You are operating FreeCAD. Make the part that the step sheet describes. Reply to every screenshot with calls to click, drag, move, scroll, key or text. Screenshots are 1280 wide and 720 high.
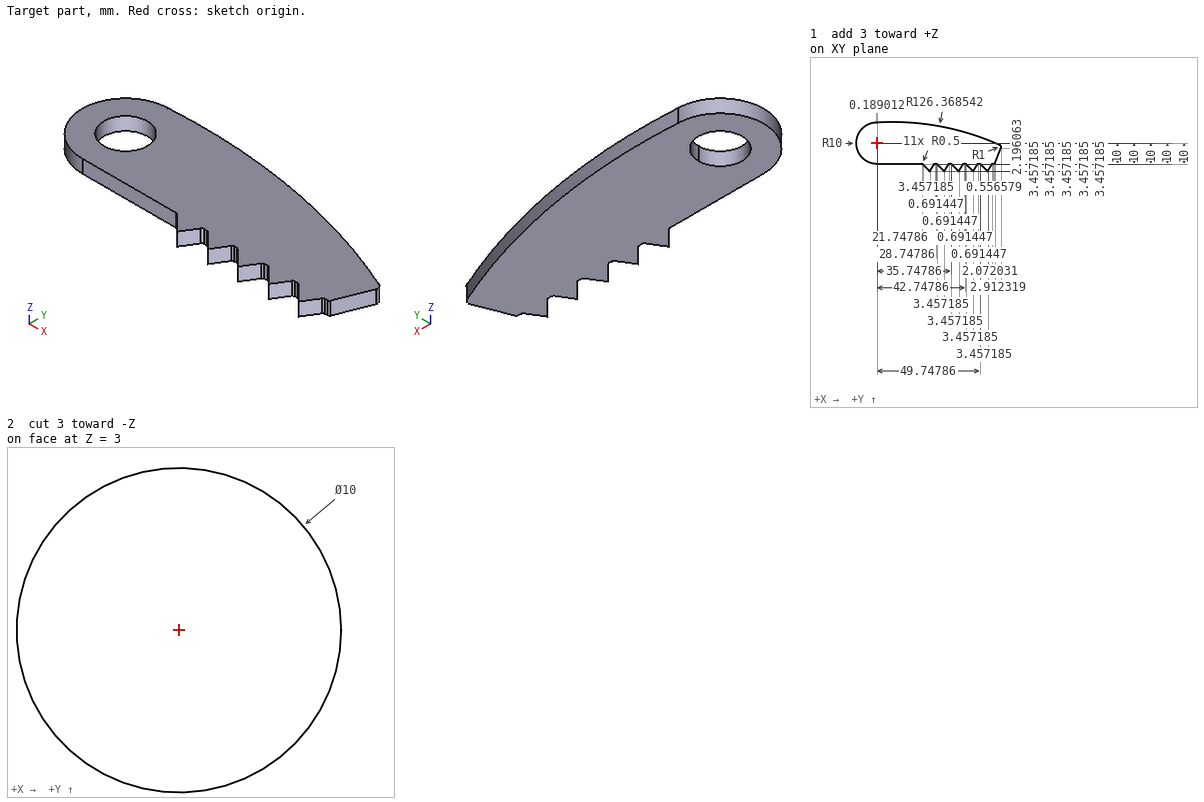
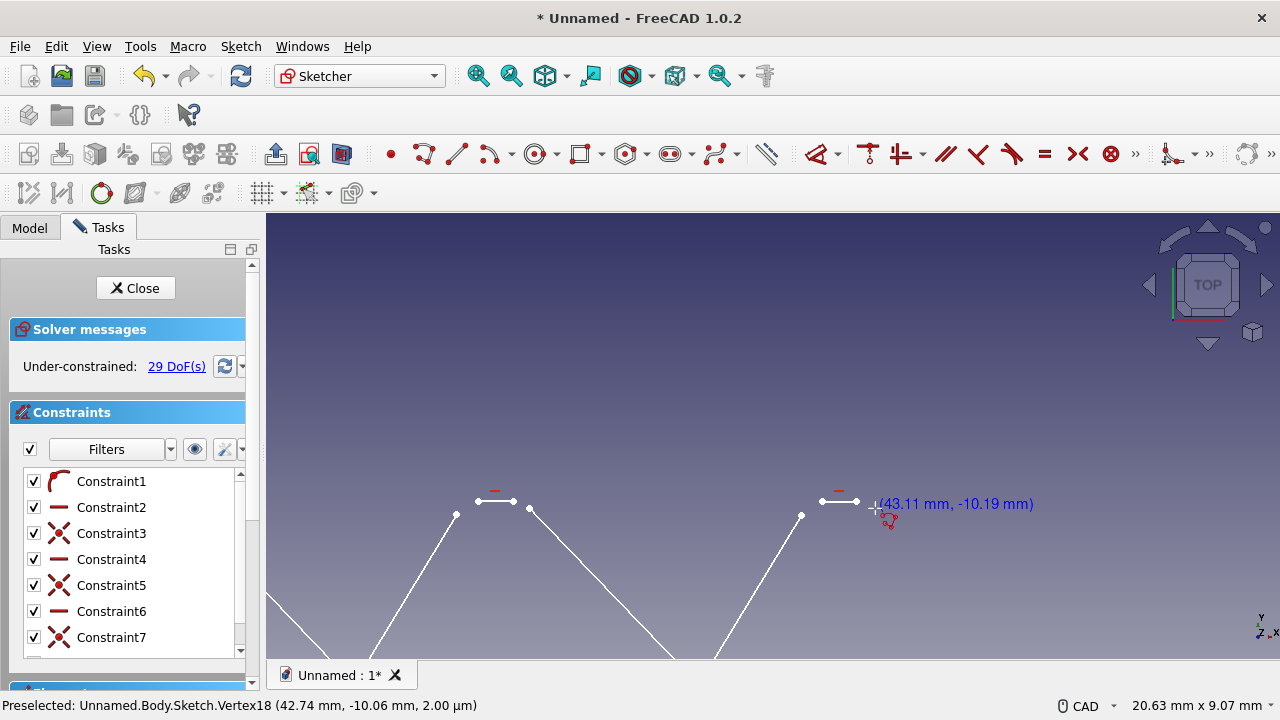
click(874, 507)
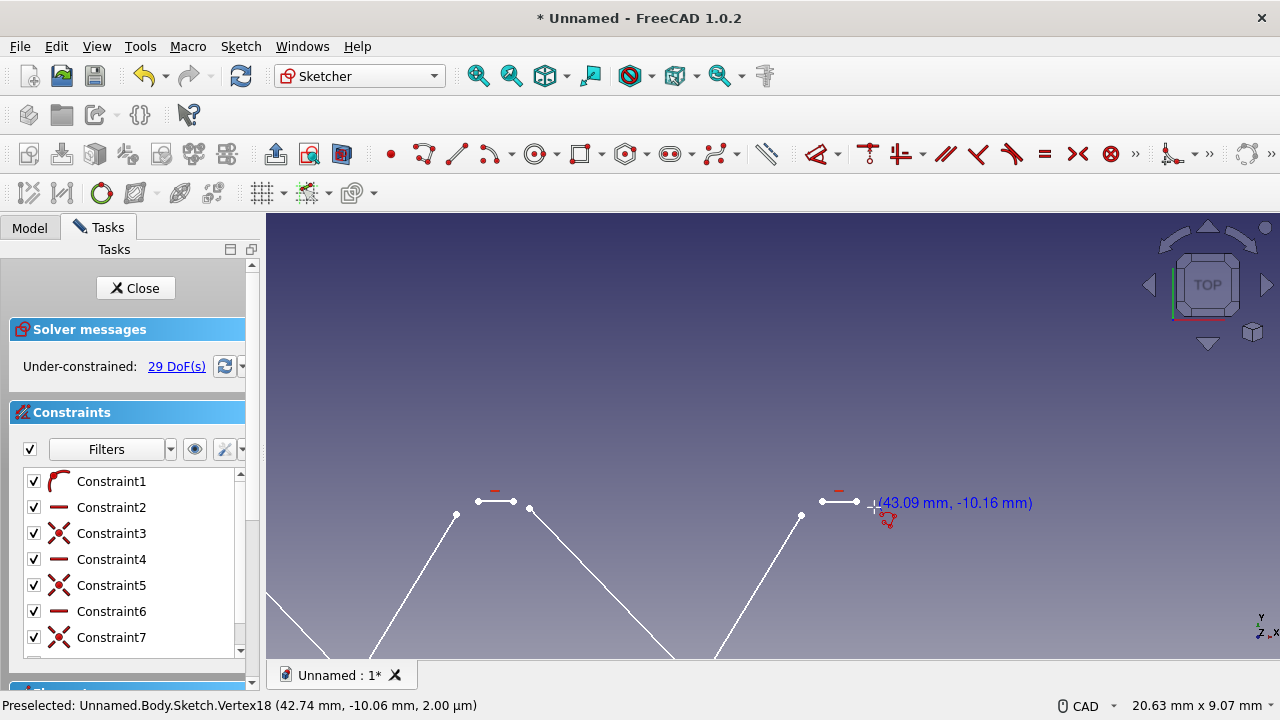
scroll(847, 503, down, 9)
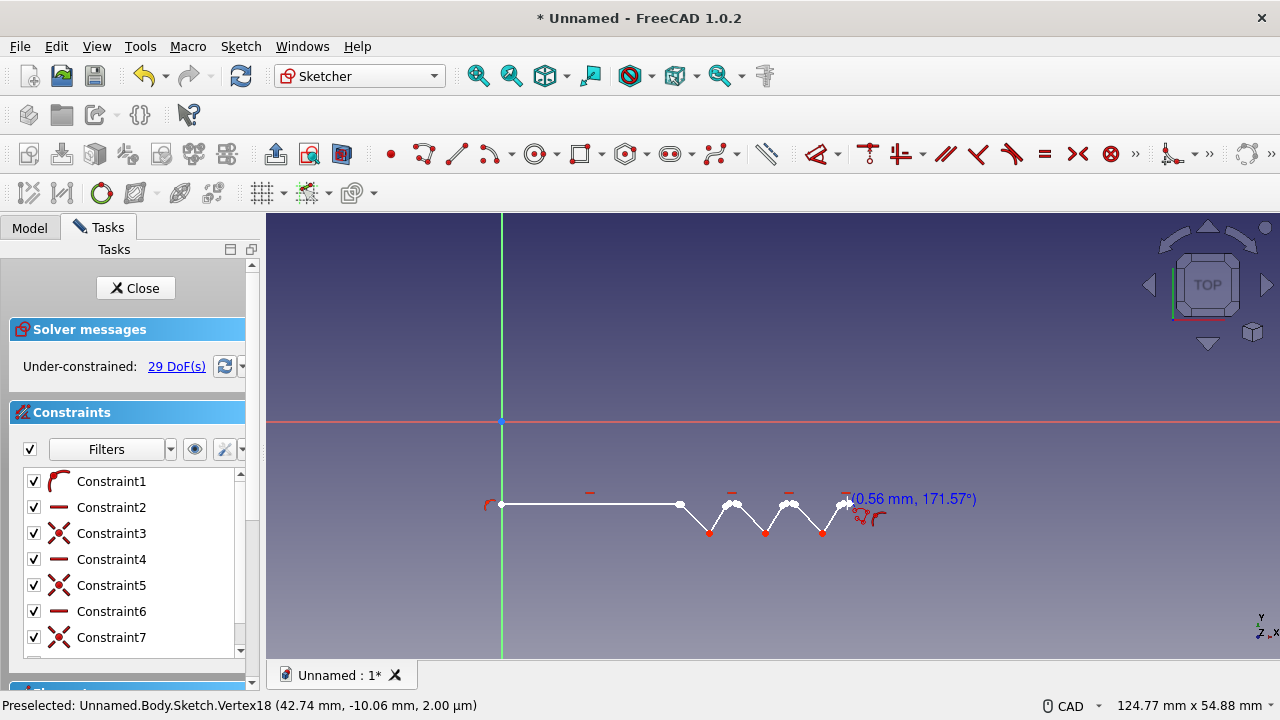
click(880, 532)
click(897, 505)
right_click(897, 505)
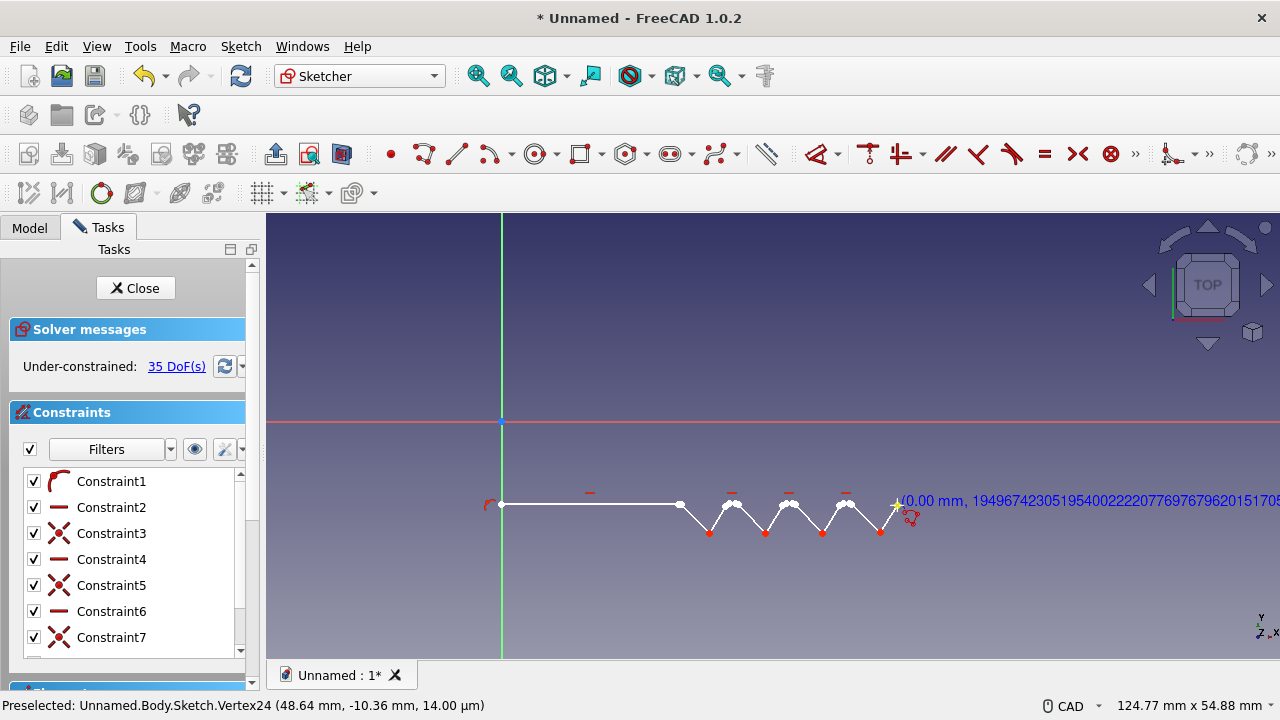
click(457, 154)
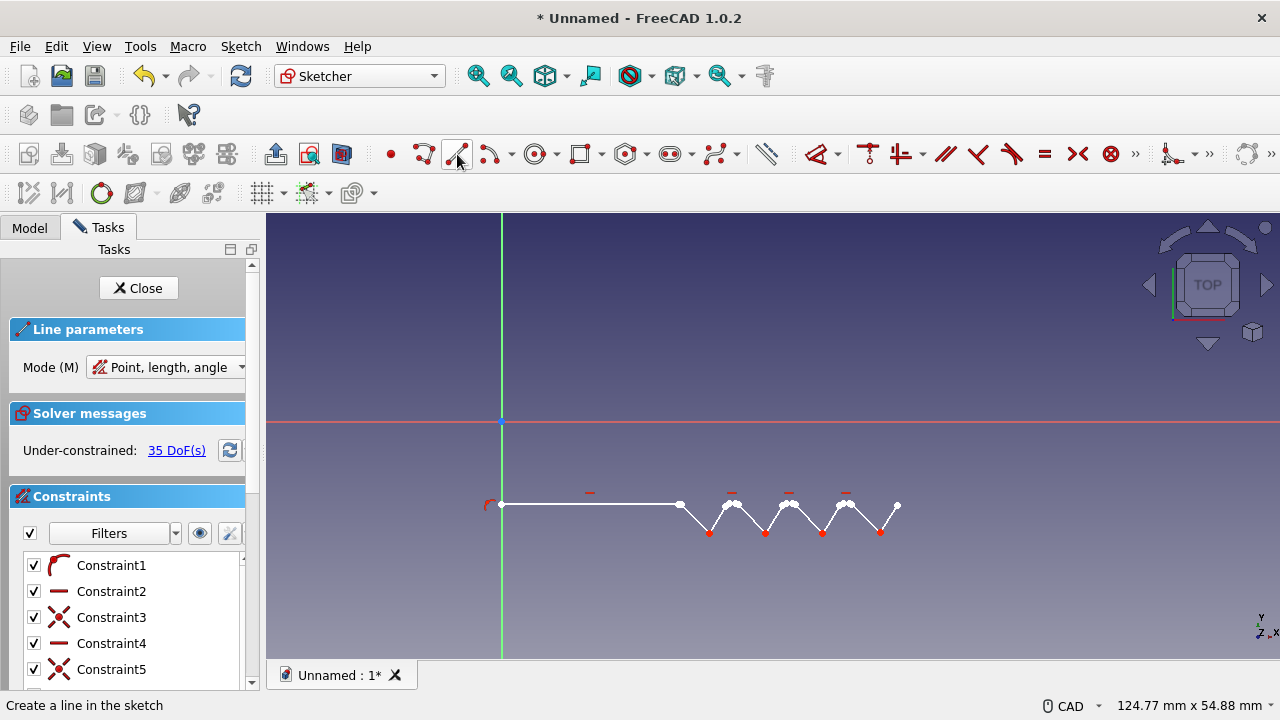
scroll(900, 503, up, 7)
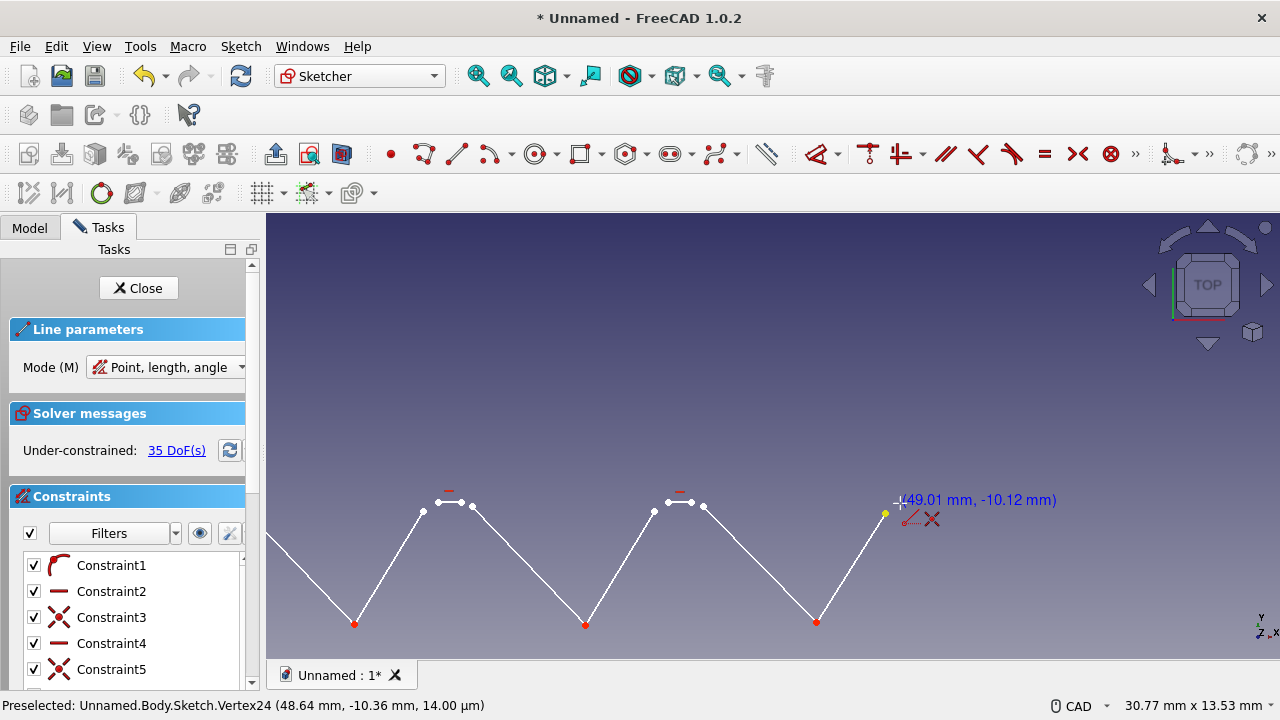
click(900, 501)
click(922, 501)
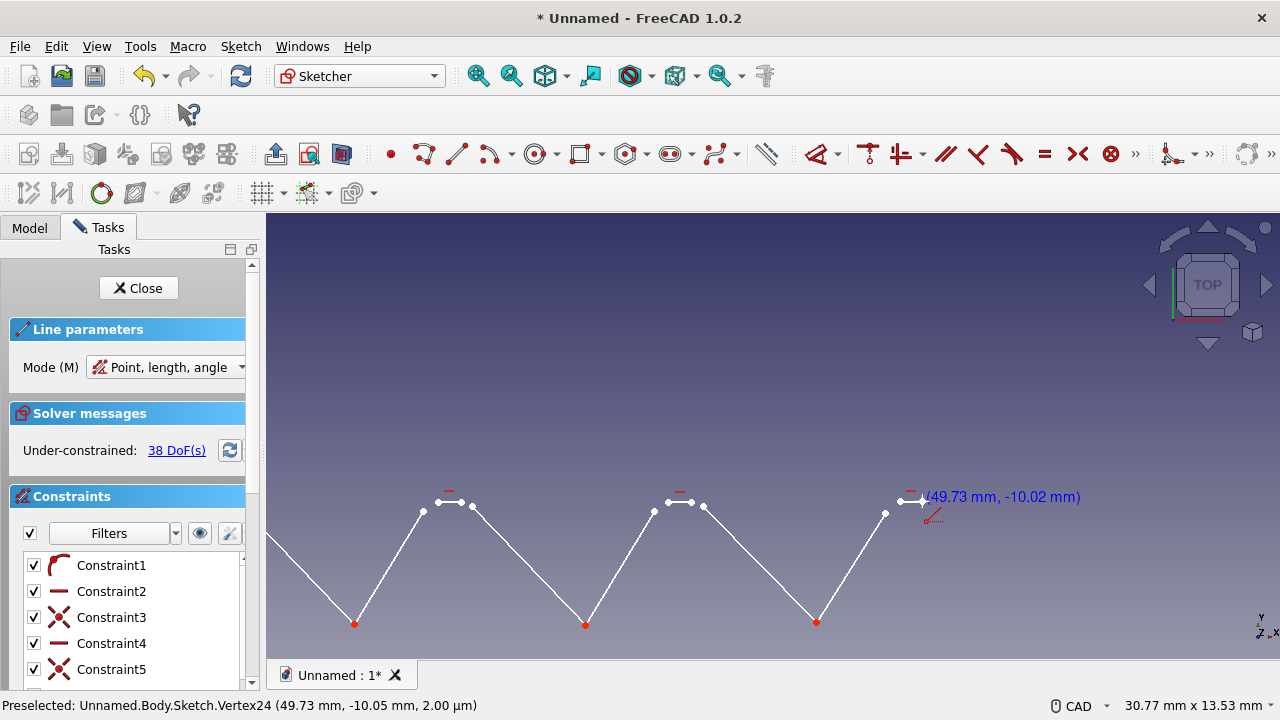
click(424, 154)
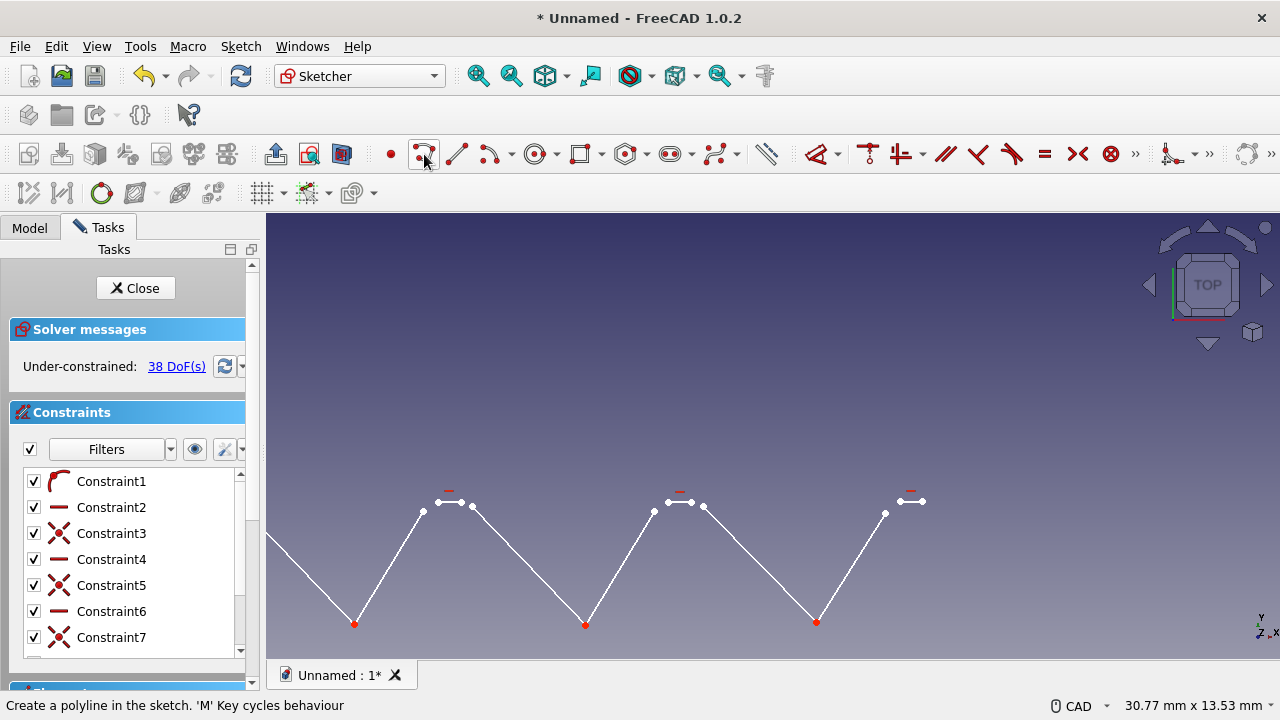
scroll(934, 506, up, 2)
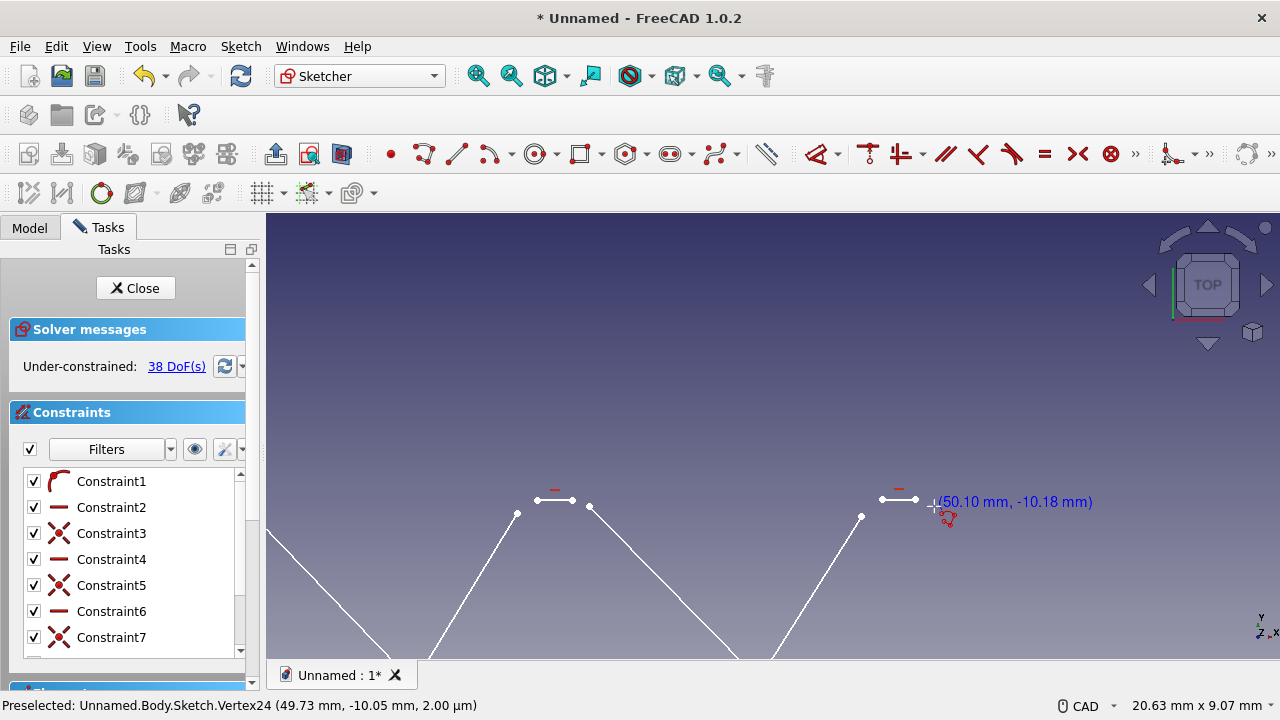
click(934, 506)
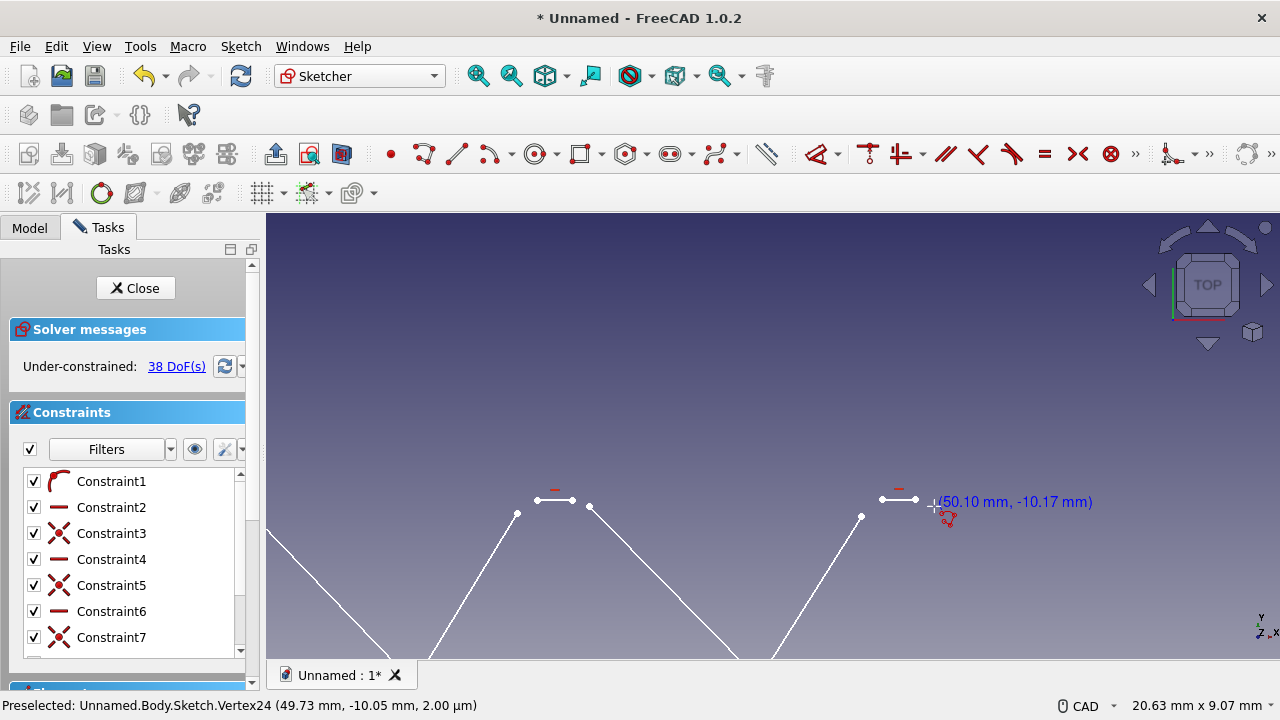
scroll(904, 503, down, 9)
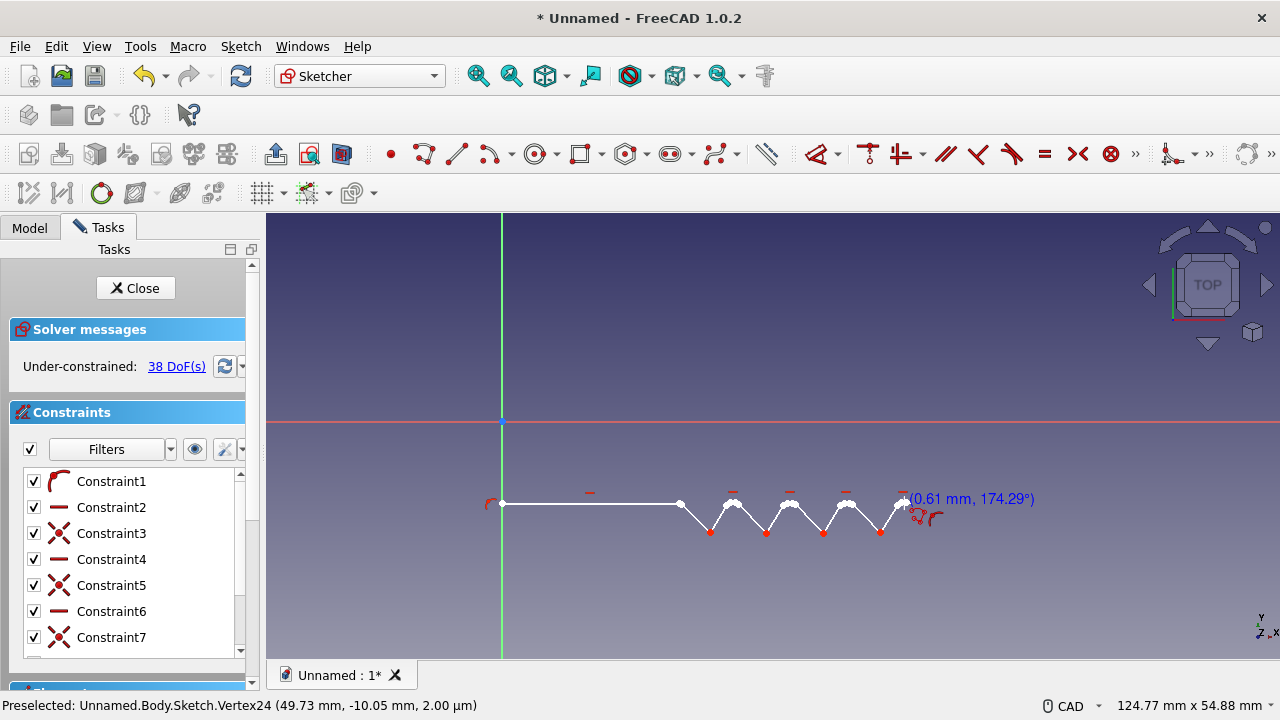
click(938, 532)
click(954, 505)
right_click(954, 505)